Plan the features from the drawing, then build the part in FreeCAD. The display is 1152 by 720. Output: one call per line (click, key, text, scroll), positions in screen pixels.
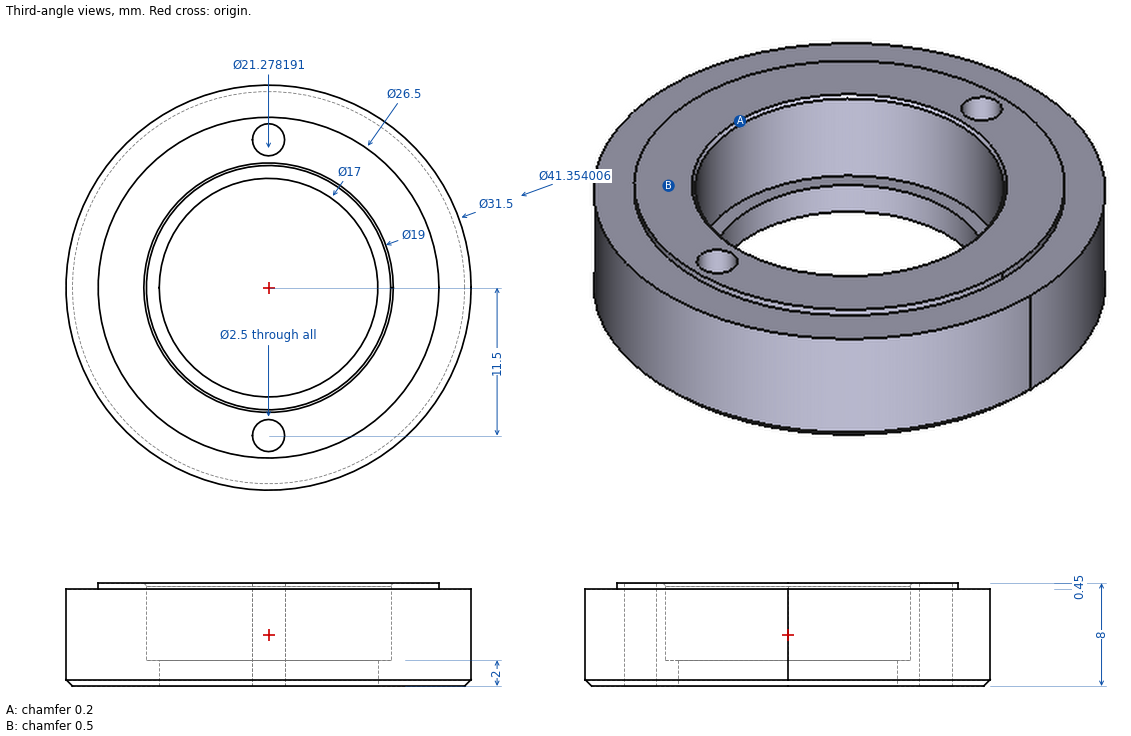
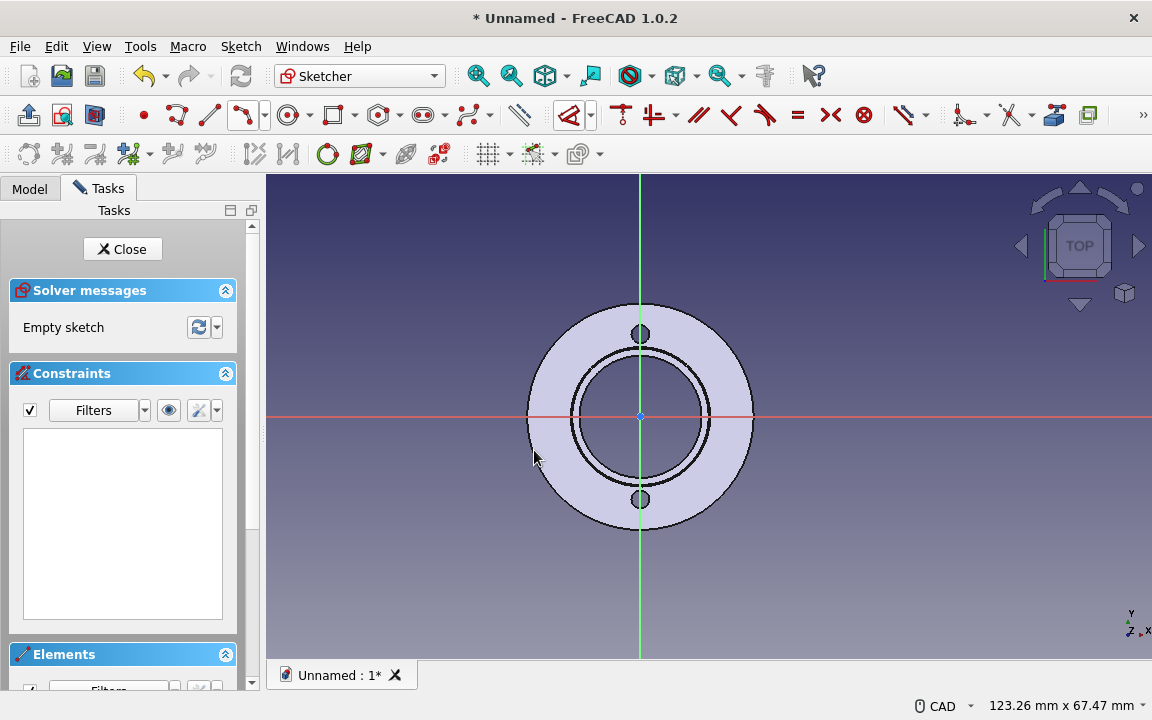
click(288, 116)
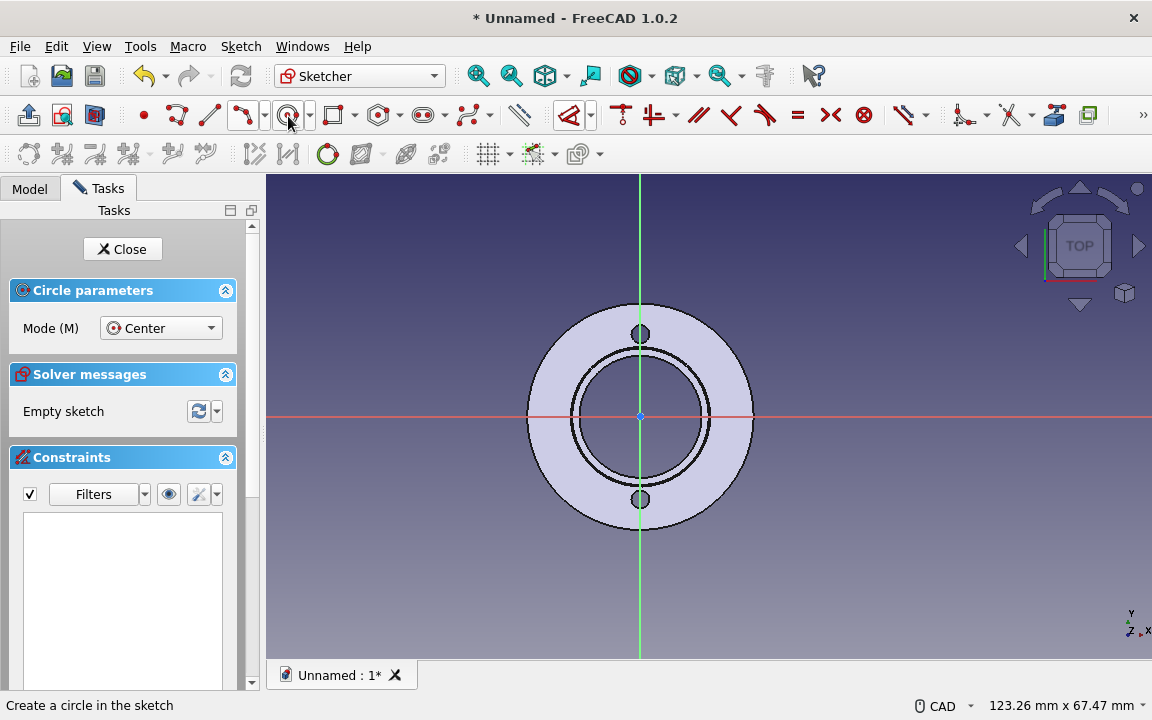
click(640, 417)
move(746, 312)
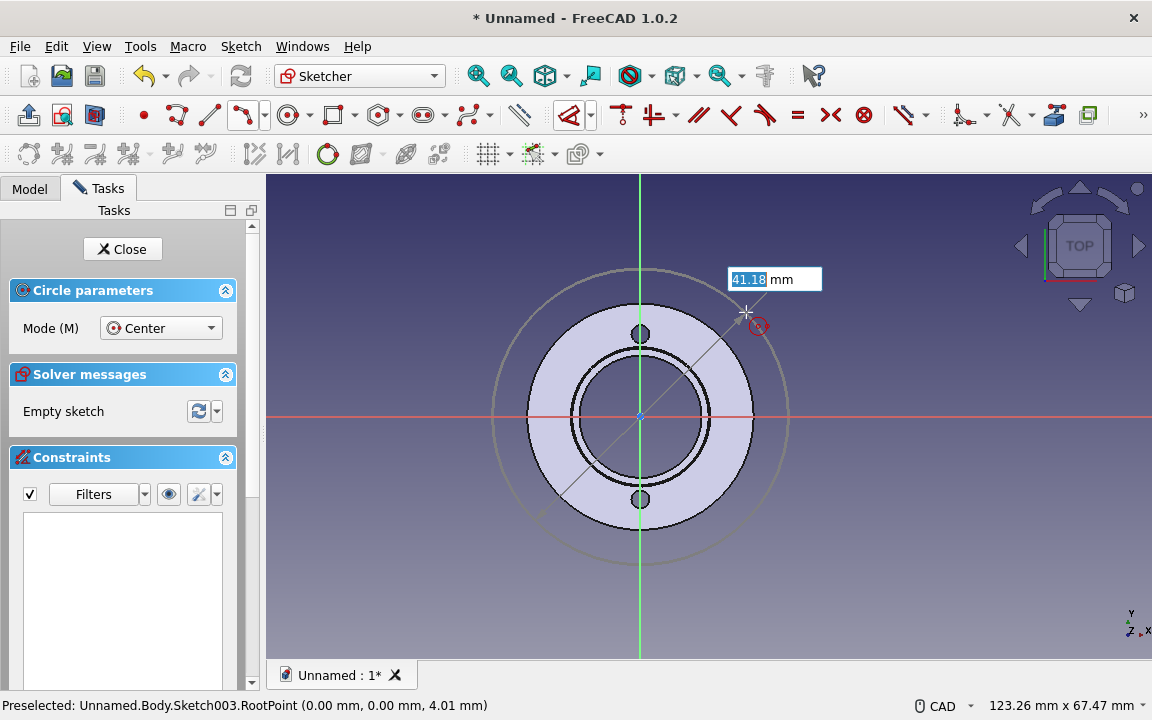
text(41.354006)
key(Return)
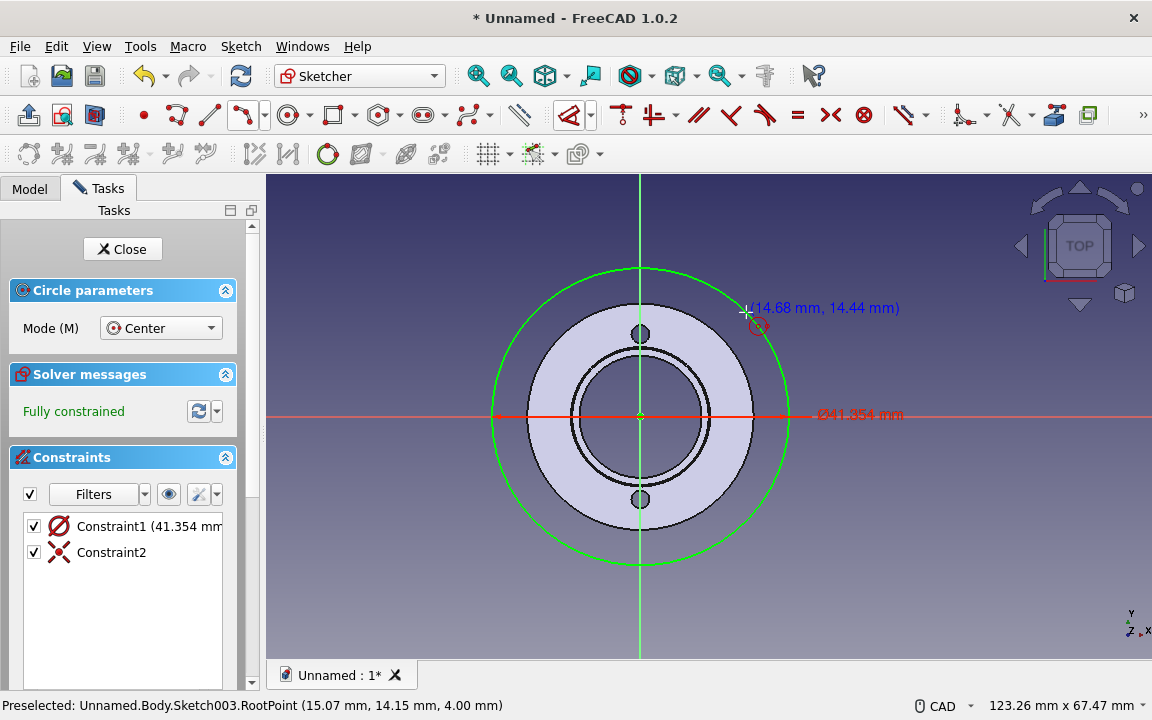
click(640, 417)
move(708, 349)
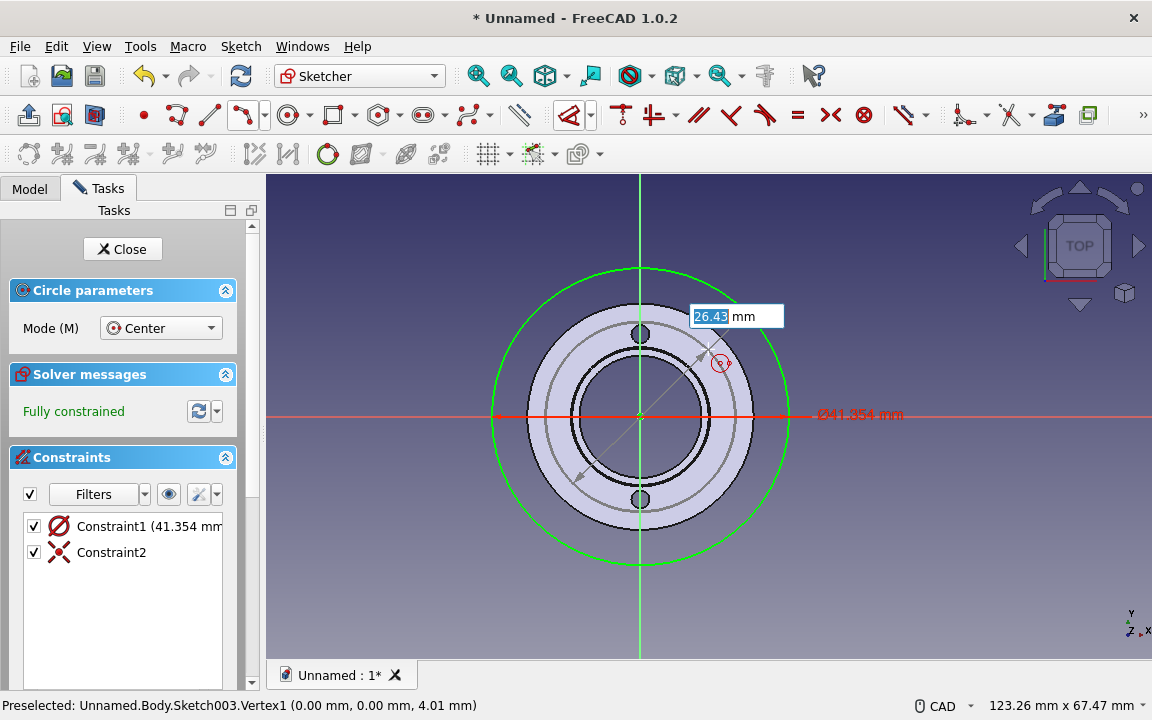
text(26.5)
key(Return)
key(Escape)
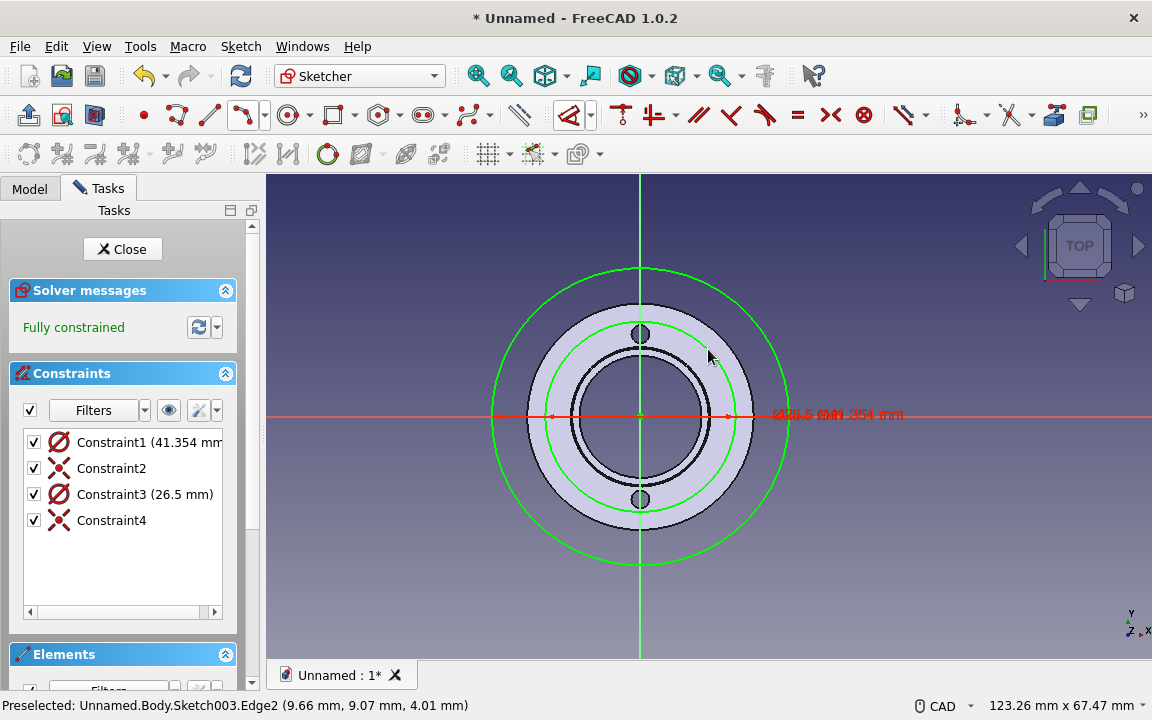
click(123, 249)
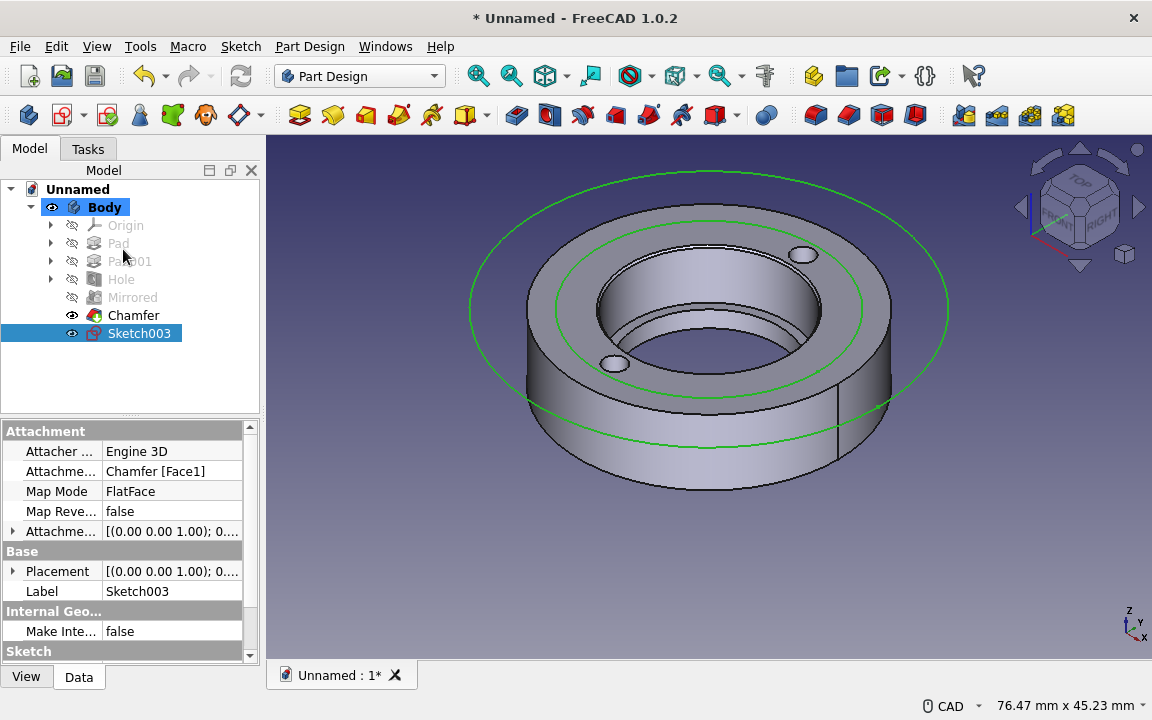
click(517, 116)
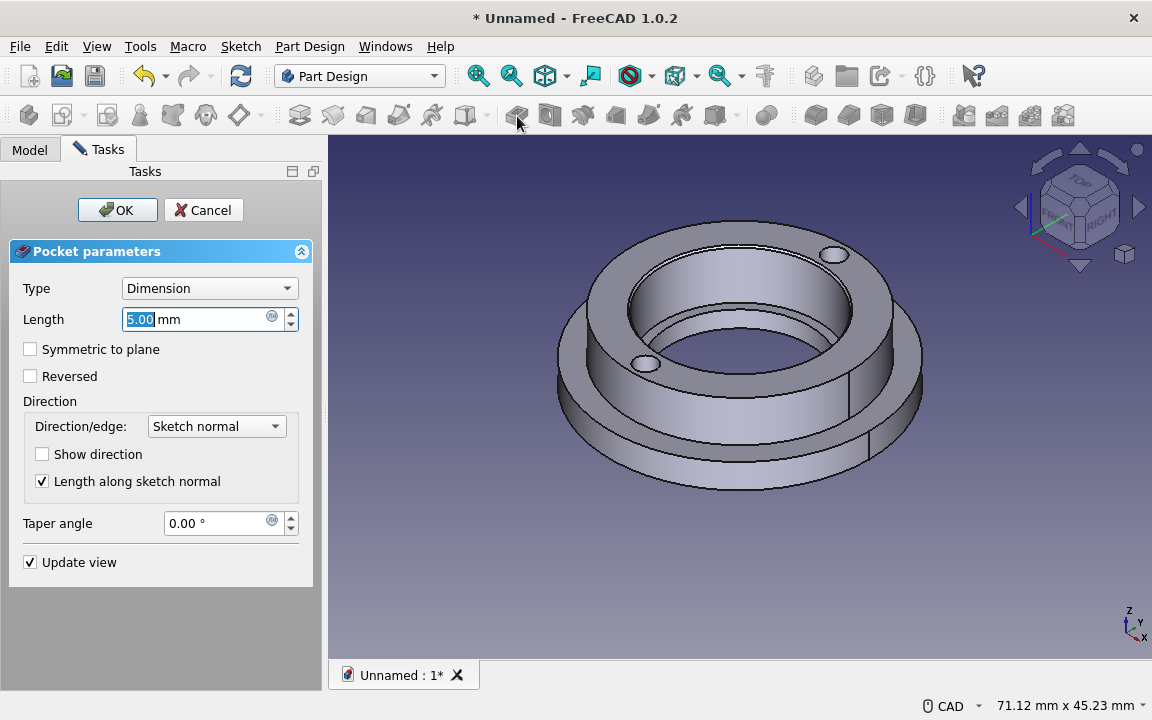
text(0.45)
key(Tab)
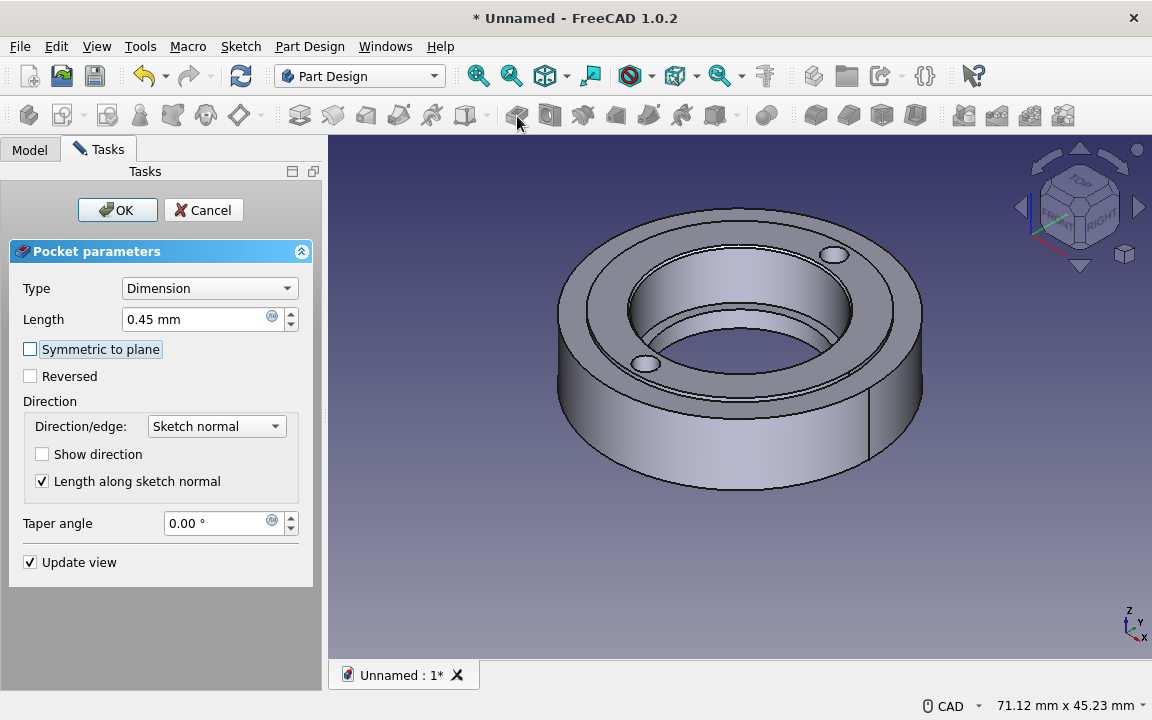
click(118, 210)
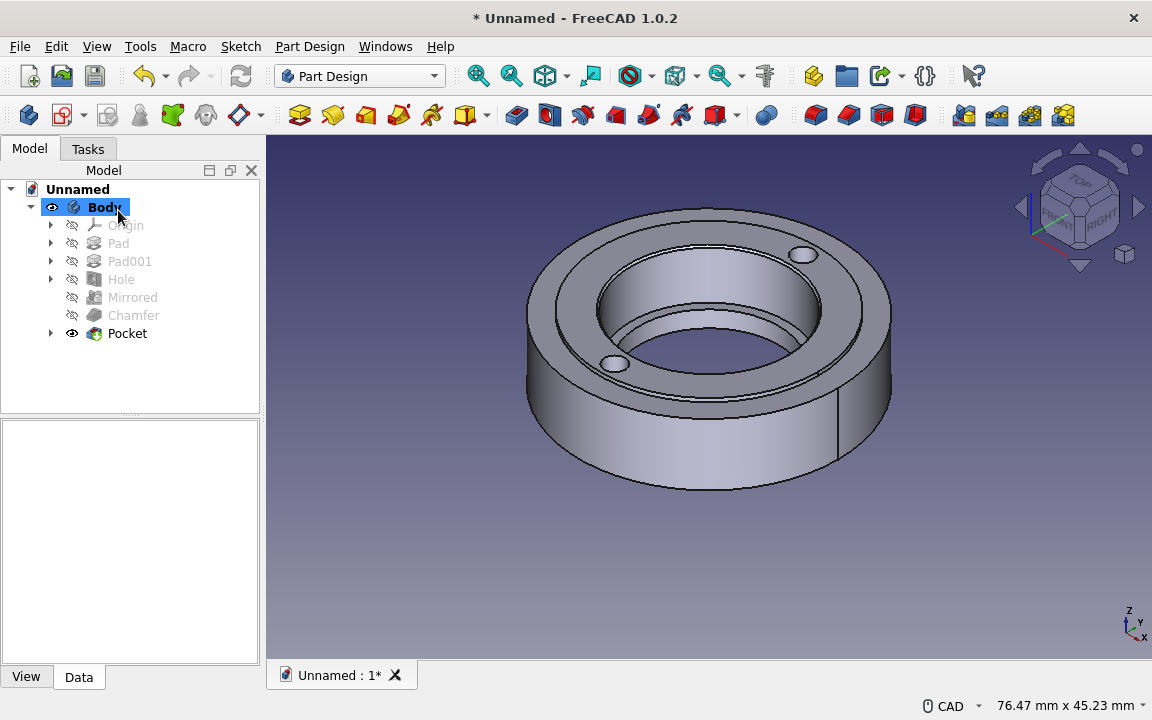
key(2)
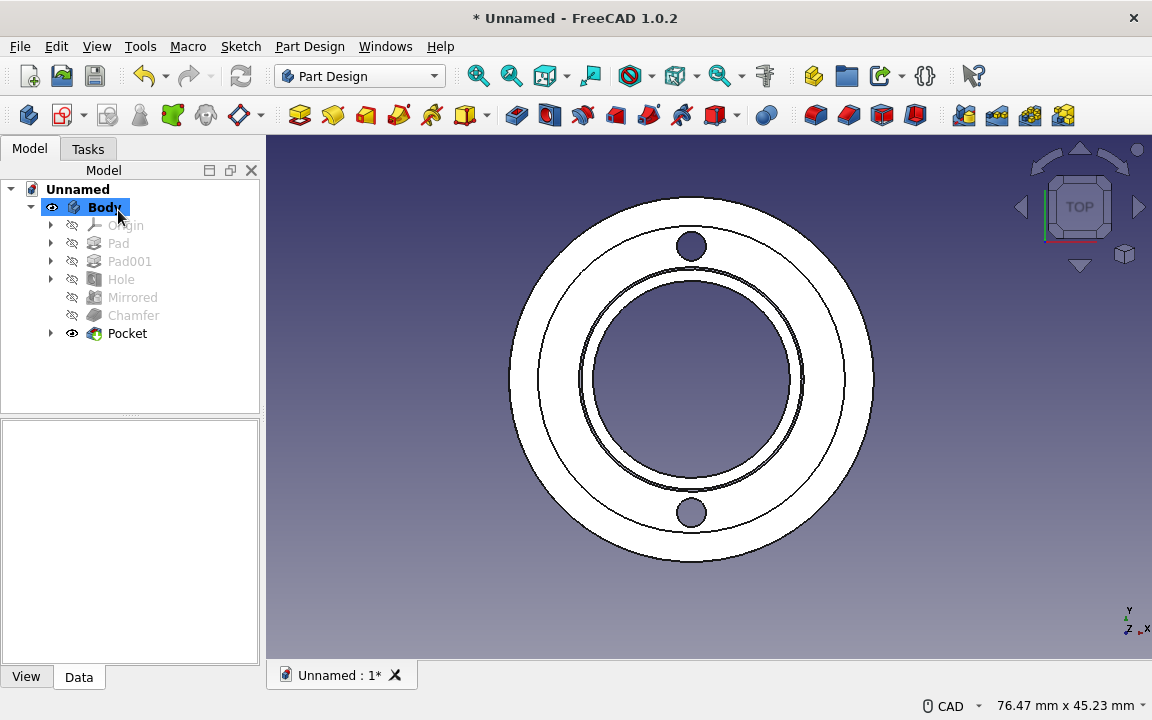
key(0)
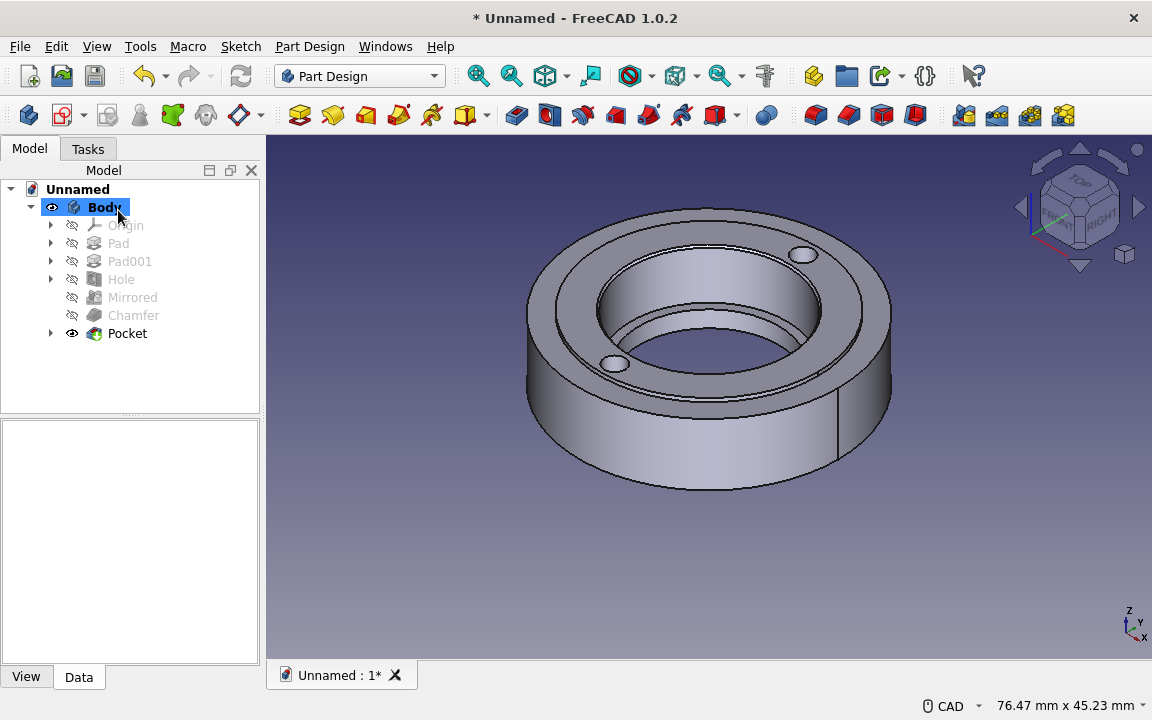
key(1)